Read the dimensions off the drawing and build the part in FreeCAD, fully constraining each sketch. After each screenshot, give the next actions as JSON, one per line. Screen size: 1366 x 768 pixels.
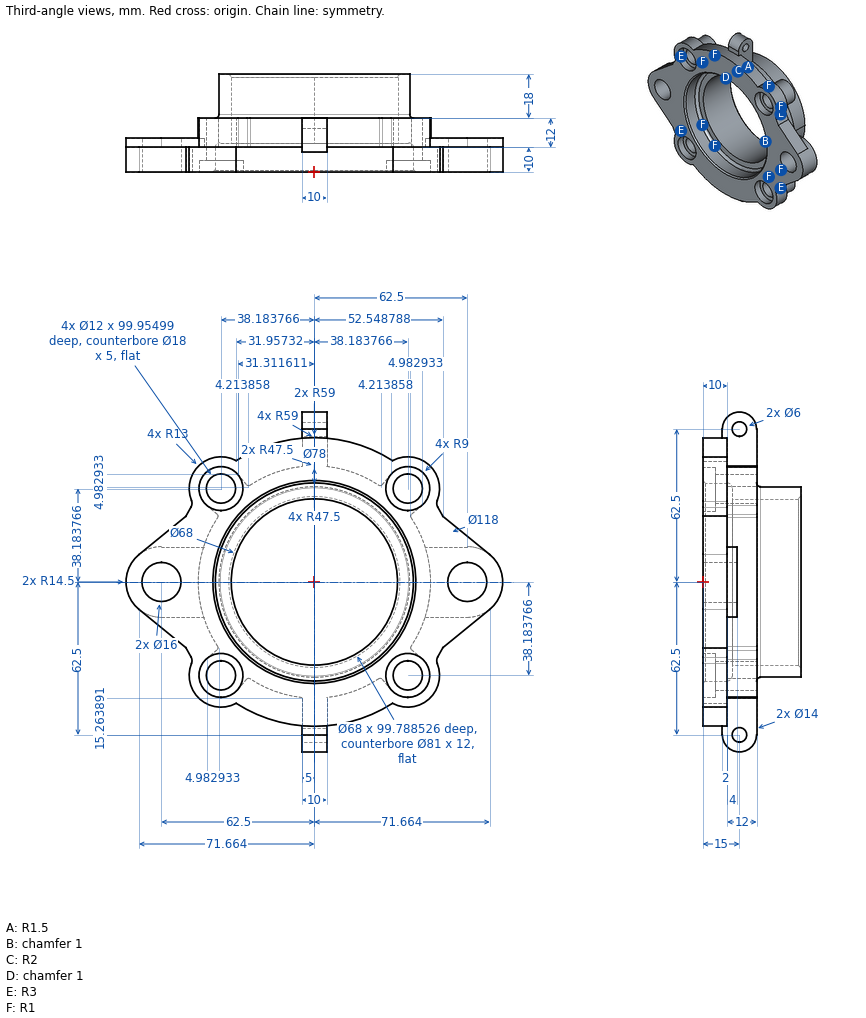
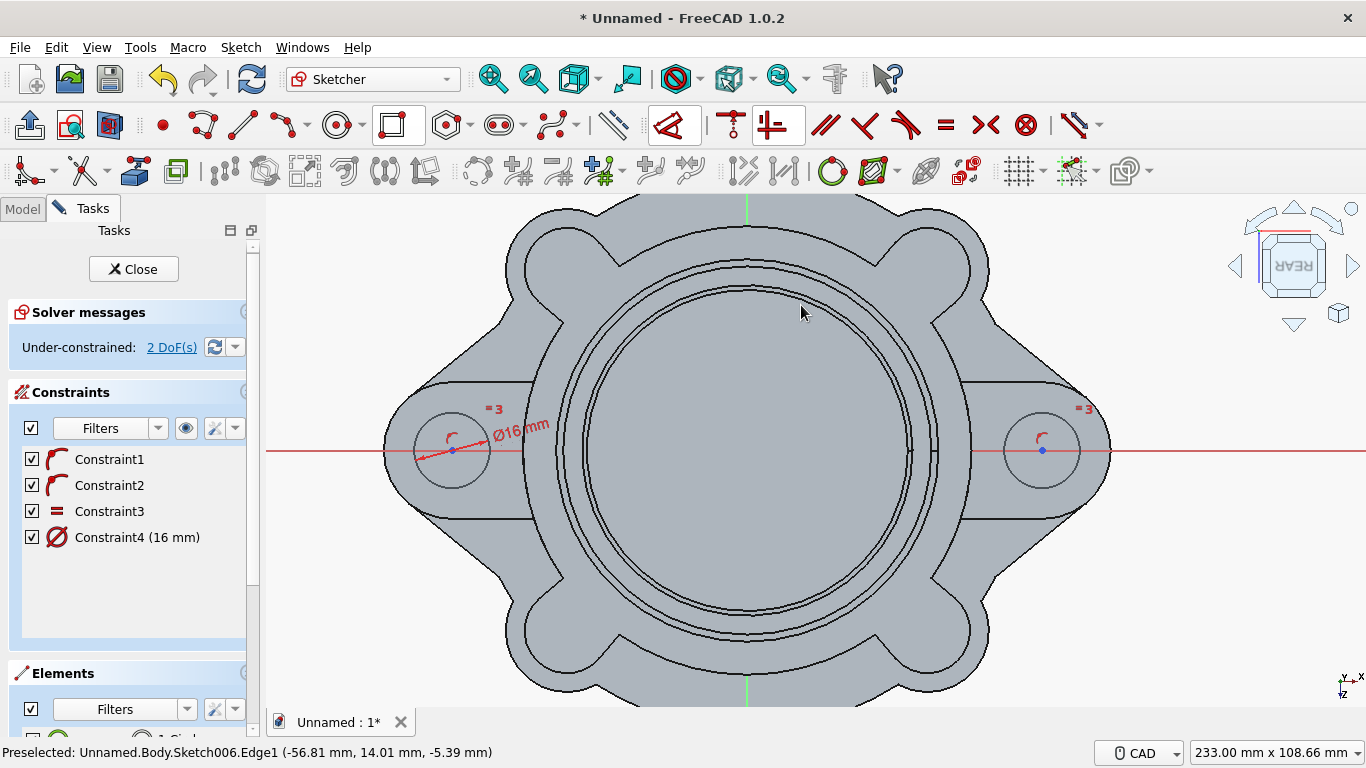
{"action": "left_click", "coordinate": [452, 450]}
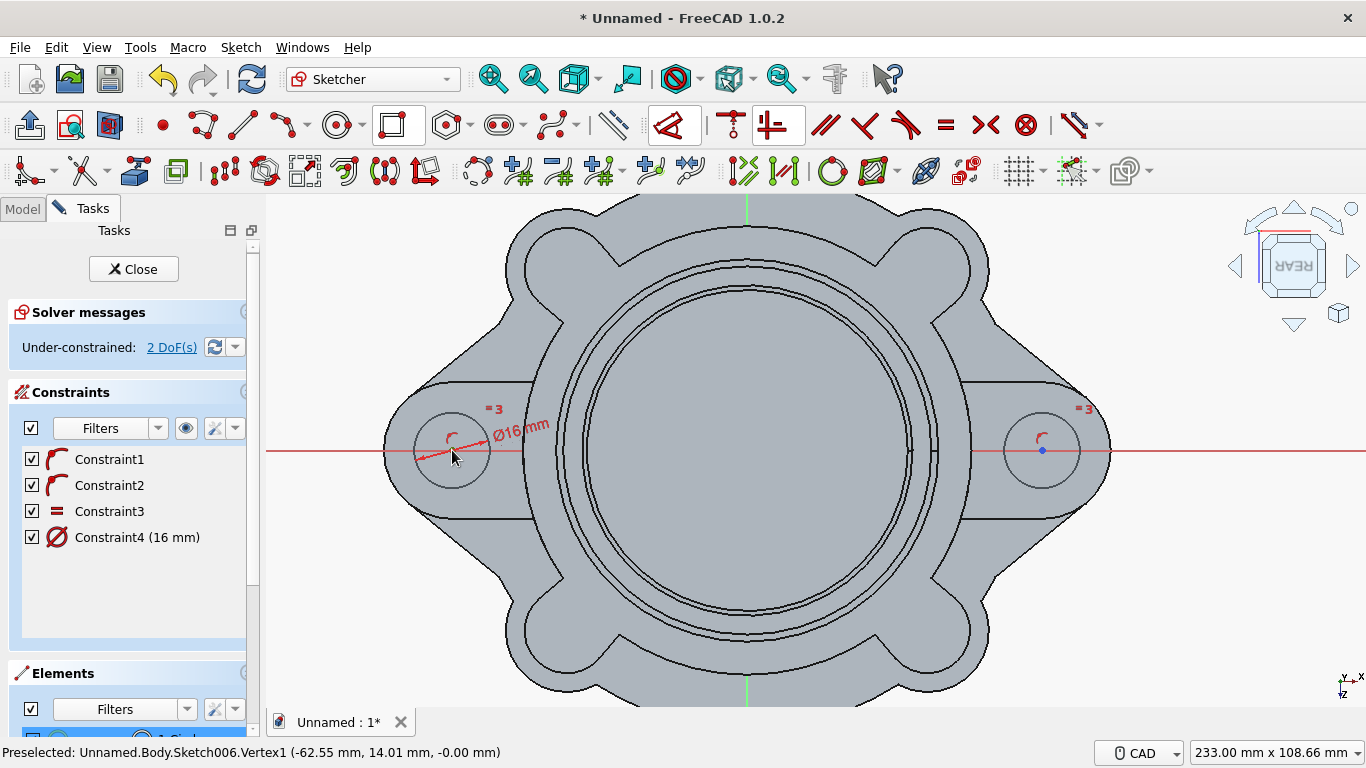
{"action": "left_click", "coordinate": [696, 126]}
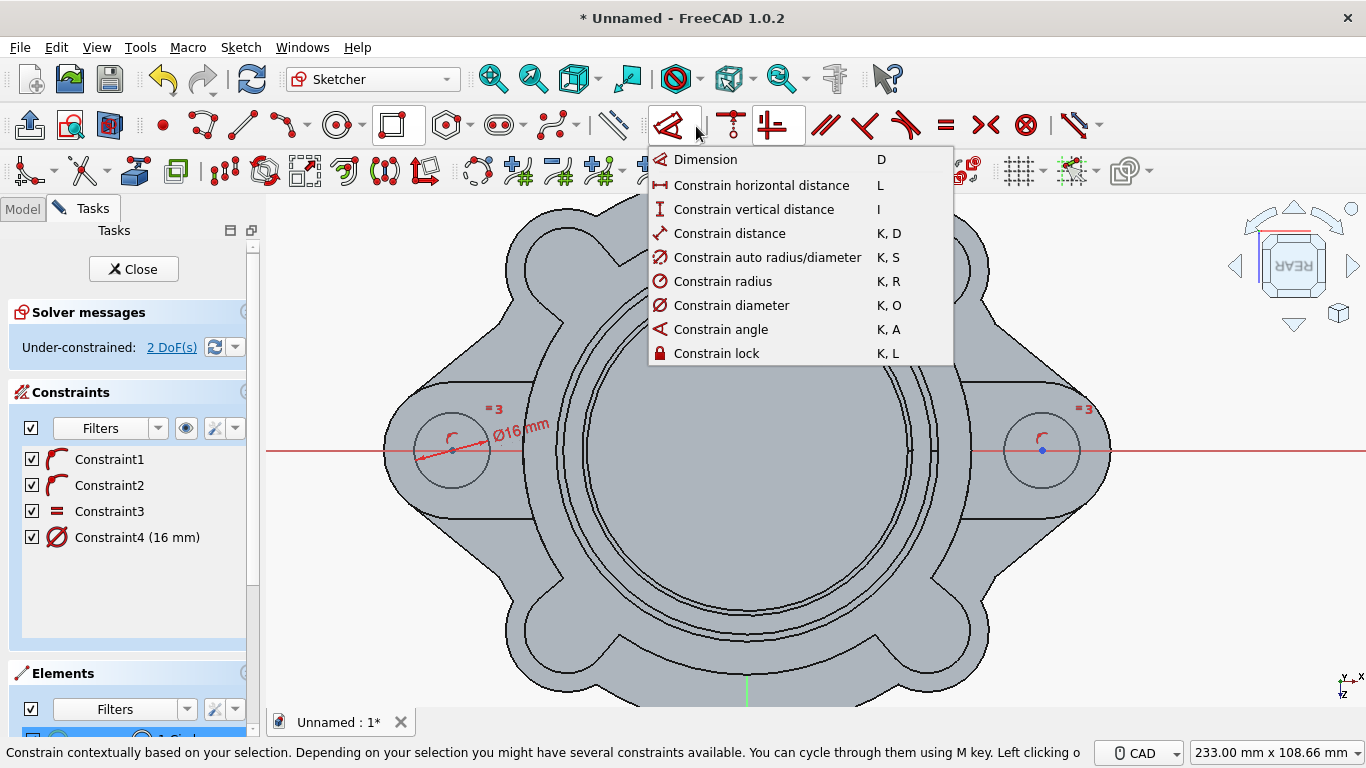
{"action": "left_click", "coordinate": [801, 185]}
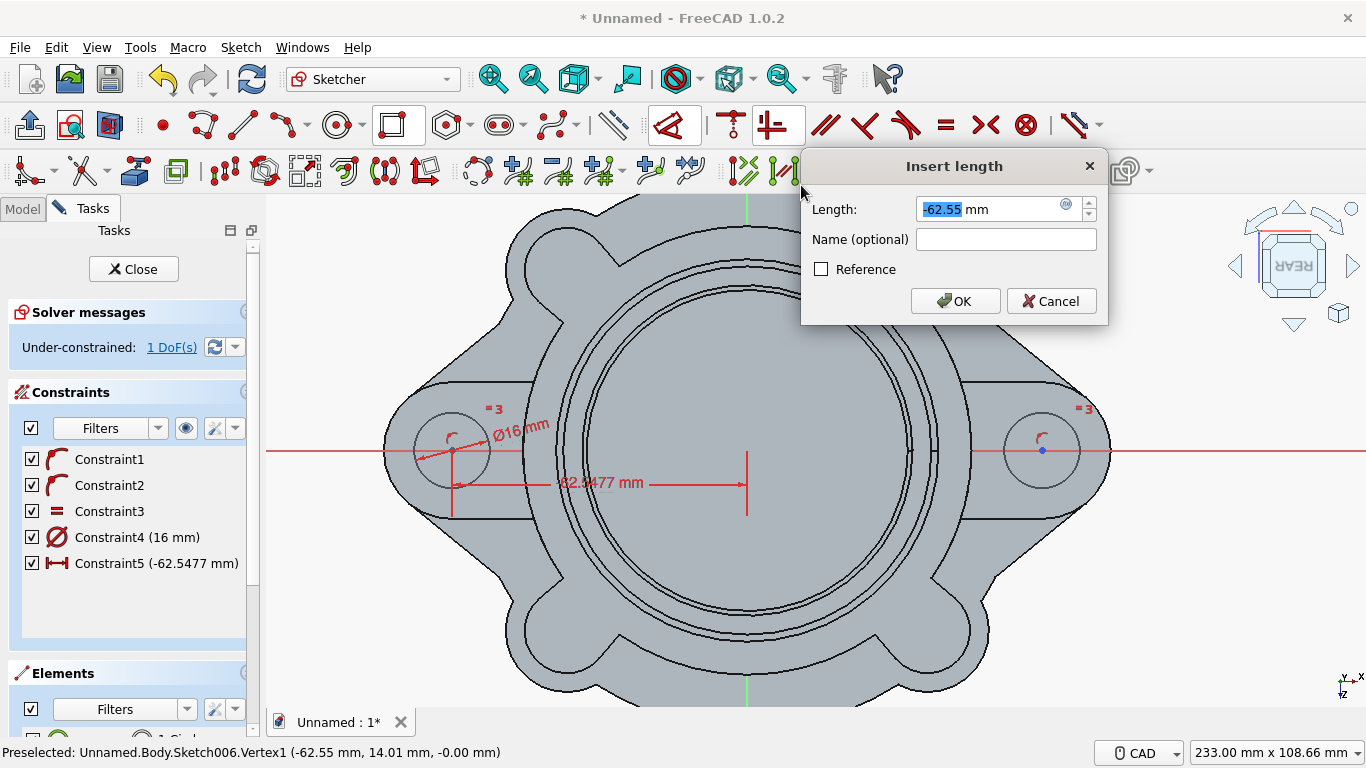
{"action": "type", "text": "-62.5"}
{"action": "key", "text": "Return"}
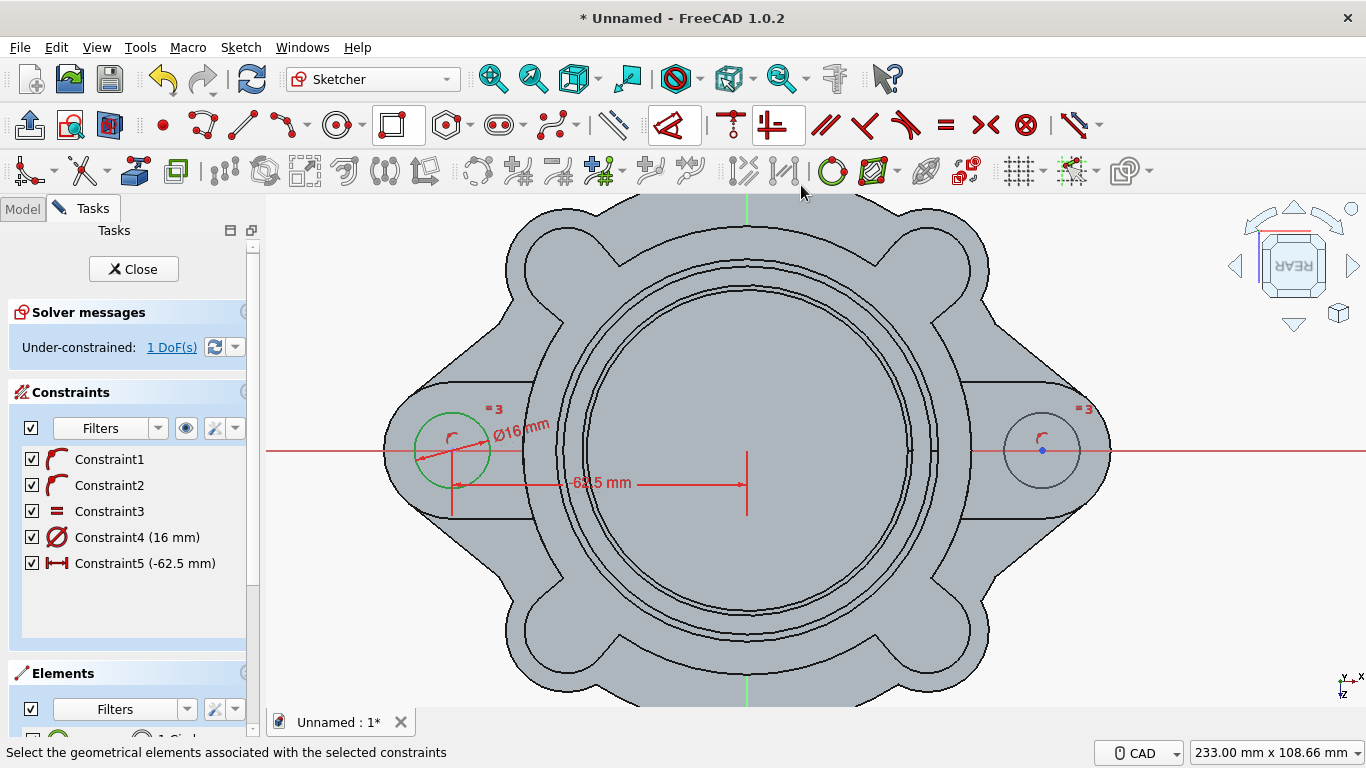
{"action": "left_click", "coordinate": [1042, 450]}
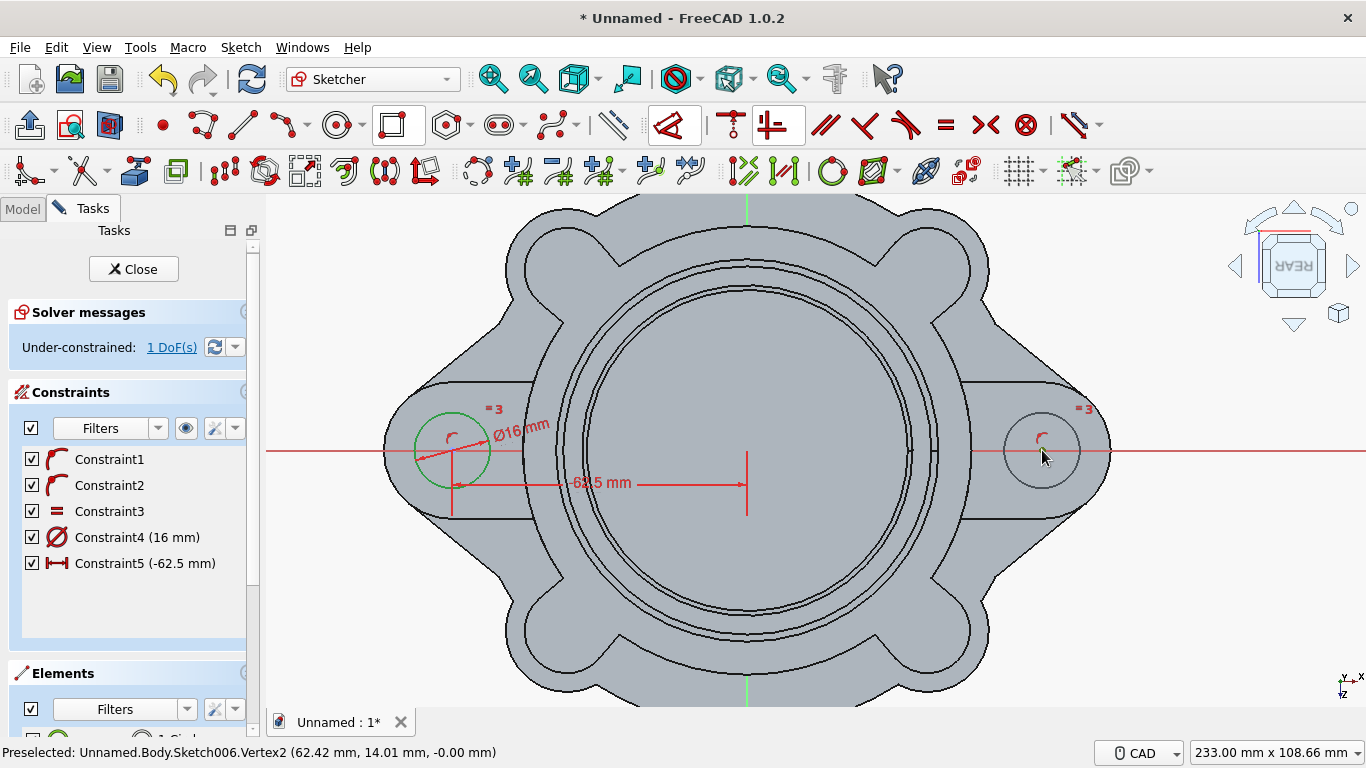
{"action": "left_click", "coordinate": [696, 126]}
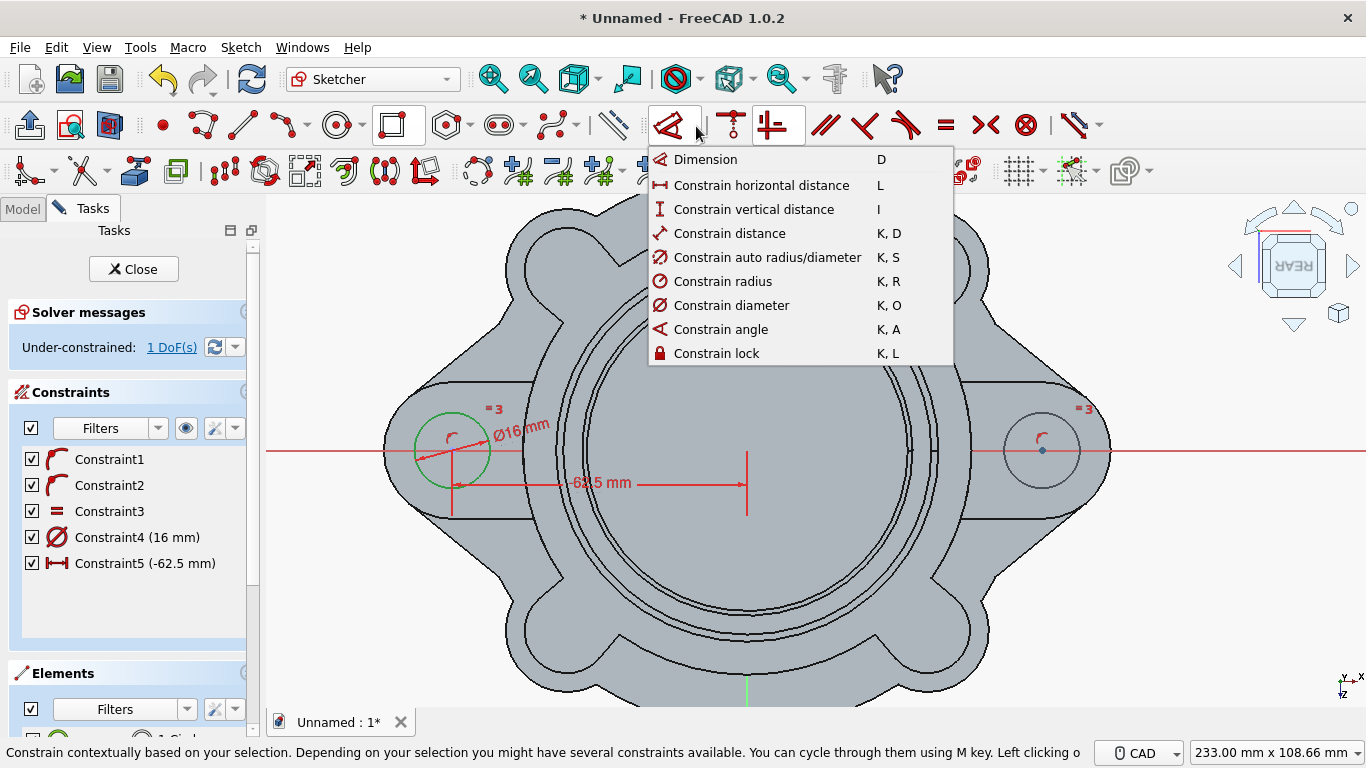
{"action": "left_click", "coordinate": [801, 185]}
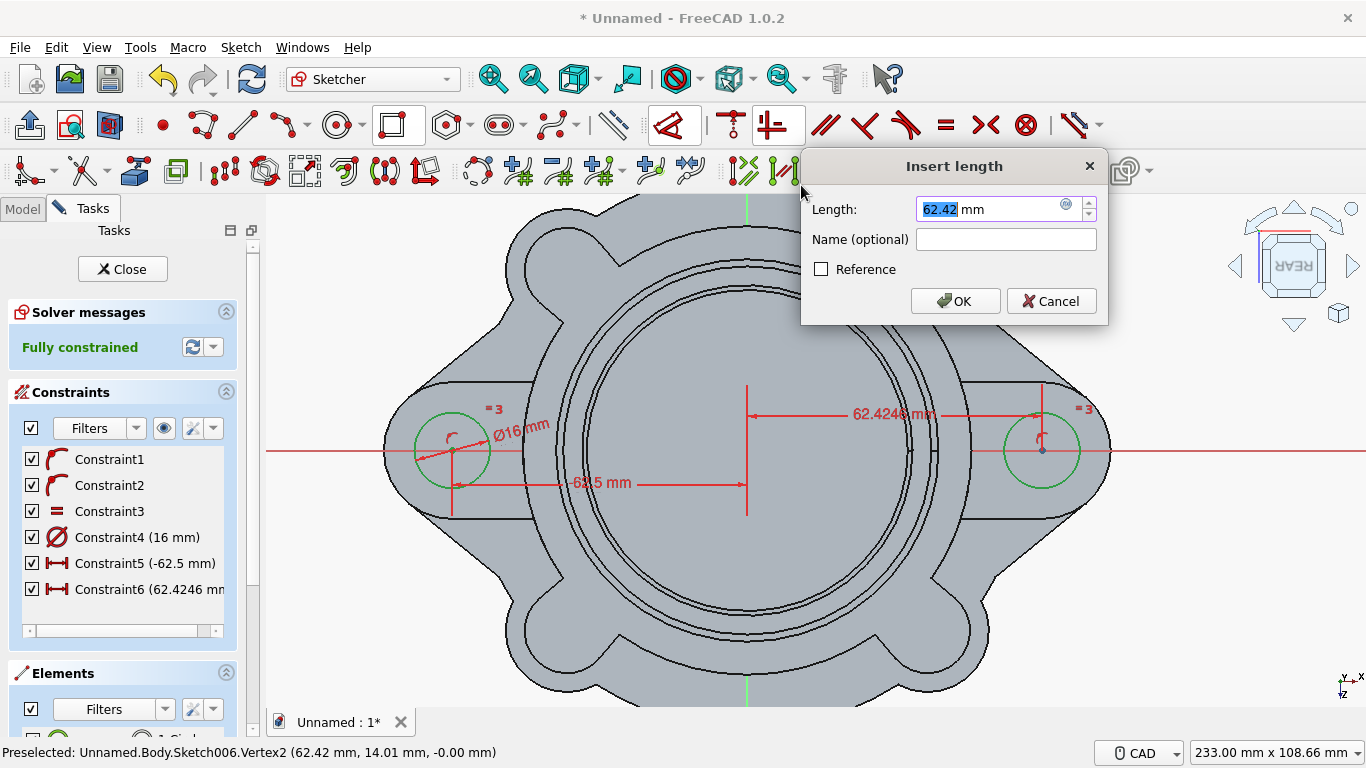
{"action": "type", "text": "62.5"}
{"action": "key", "text": "Return"}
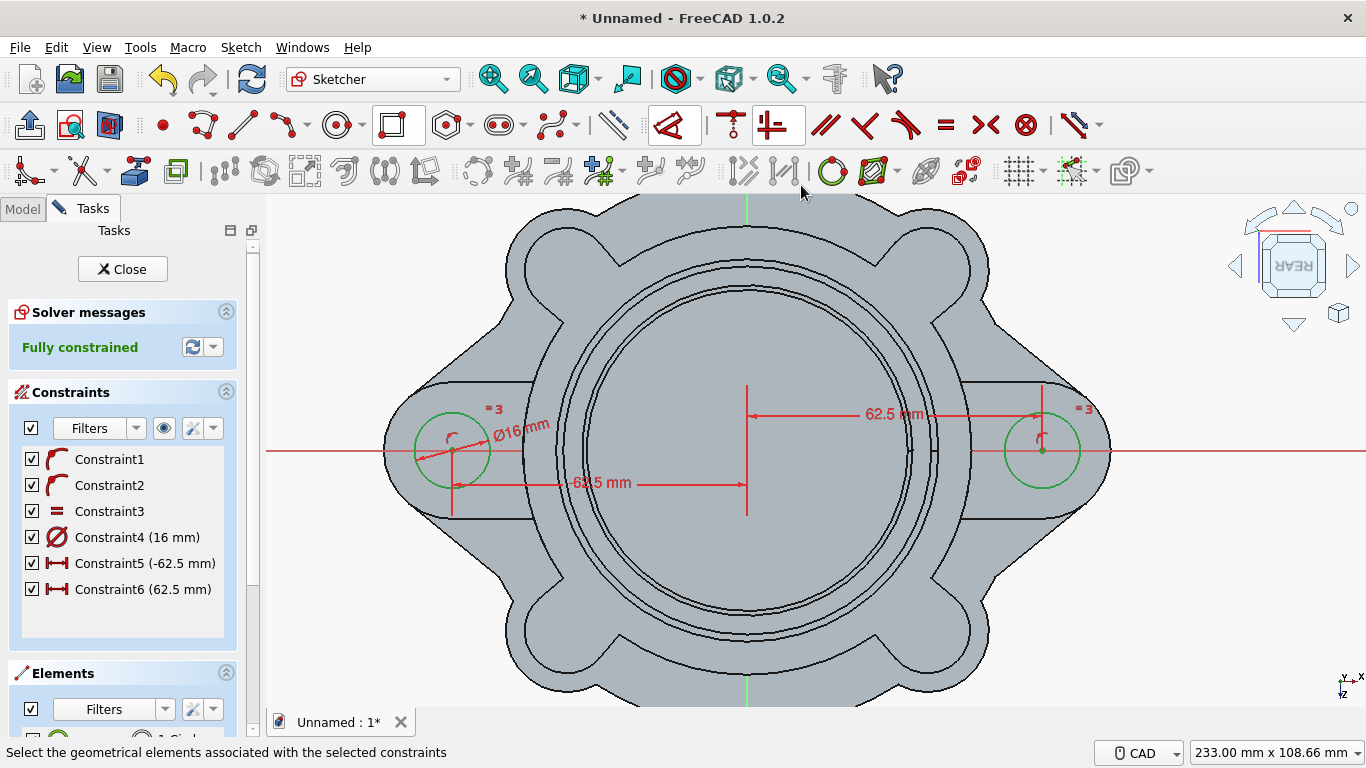
{"action": "left_click", "coordinate": [123, 269]}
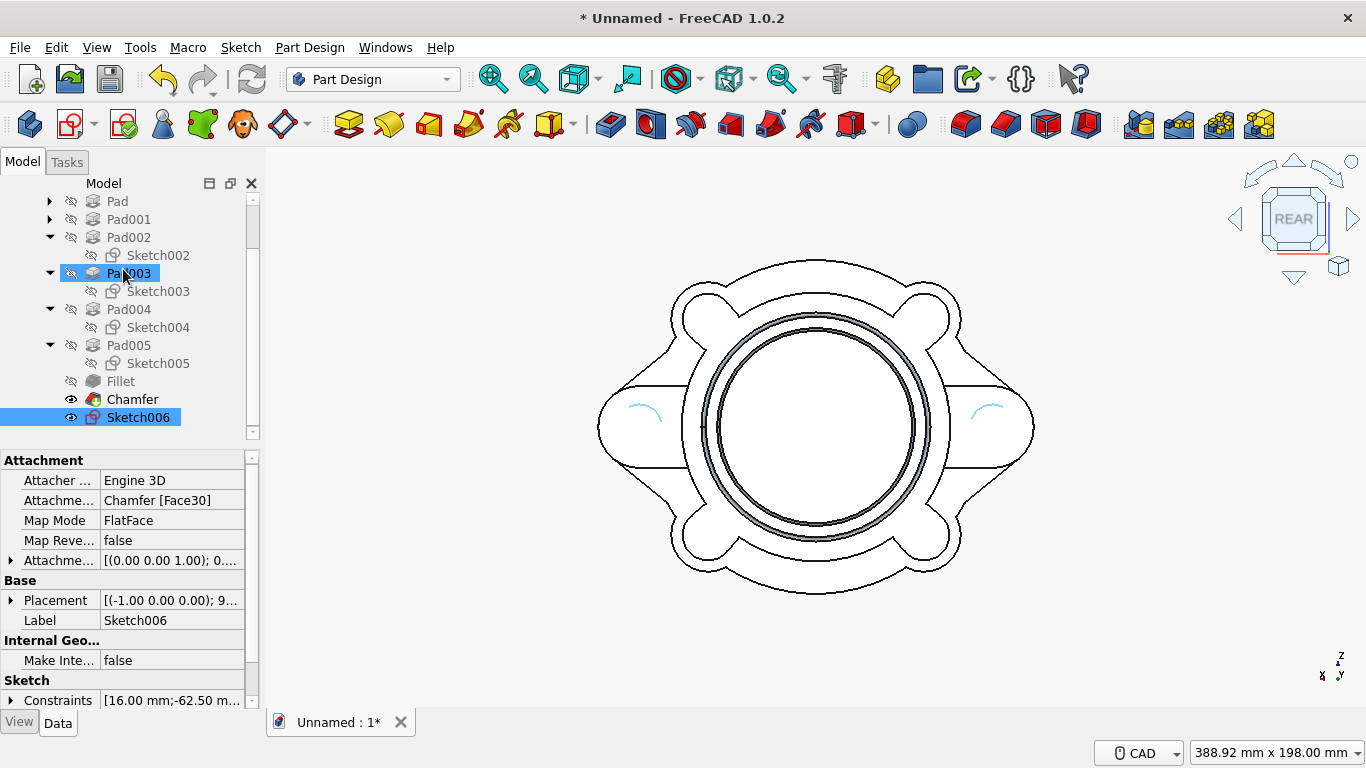
{"action": "left_click", "coordinate": [612, 124]}